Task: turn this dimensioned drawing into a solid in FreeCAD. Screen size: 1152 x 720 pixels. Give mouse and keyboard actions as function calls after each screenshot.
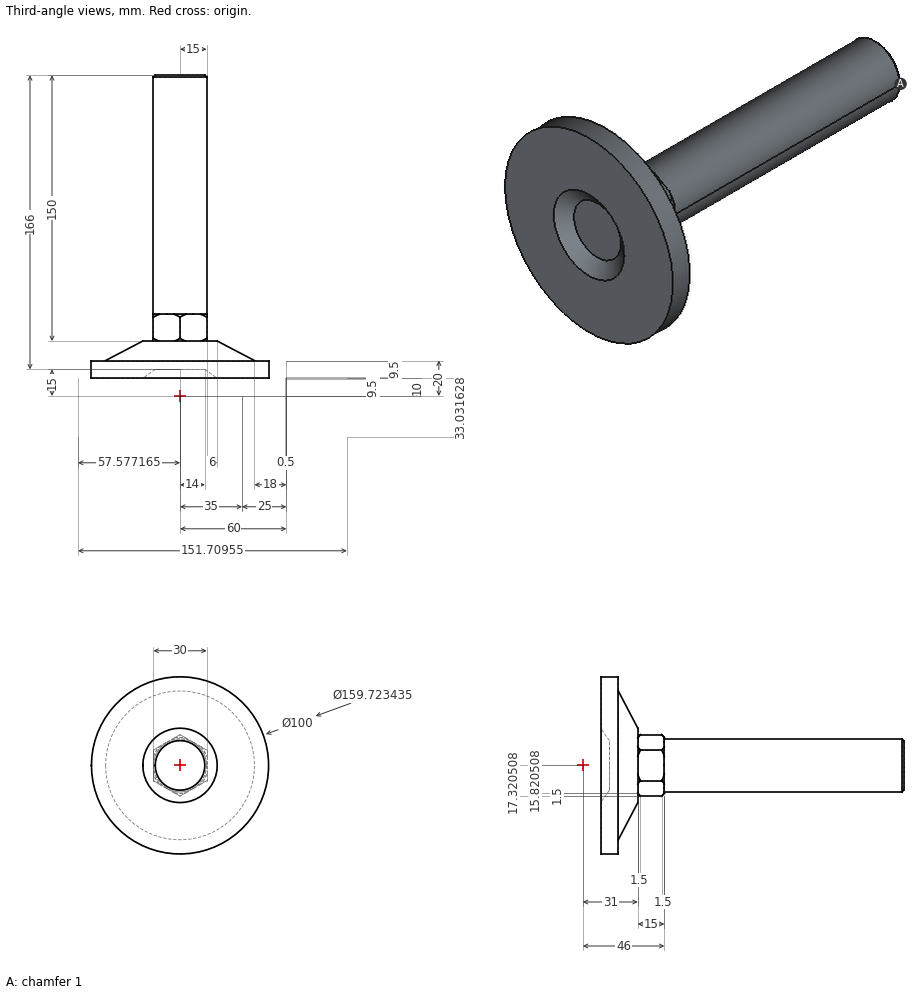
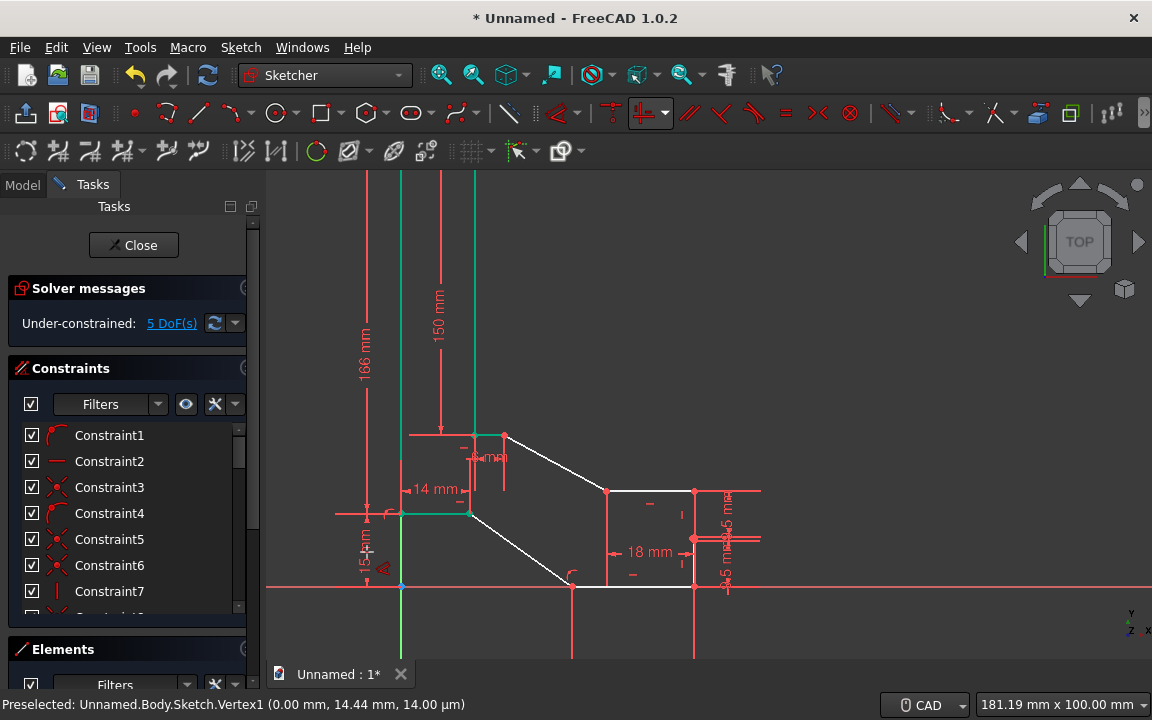
click(572, 587)
click(487, 621)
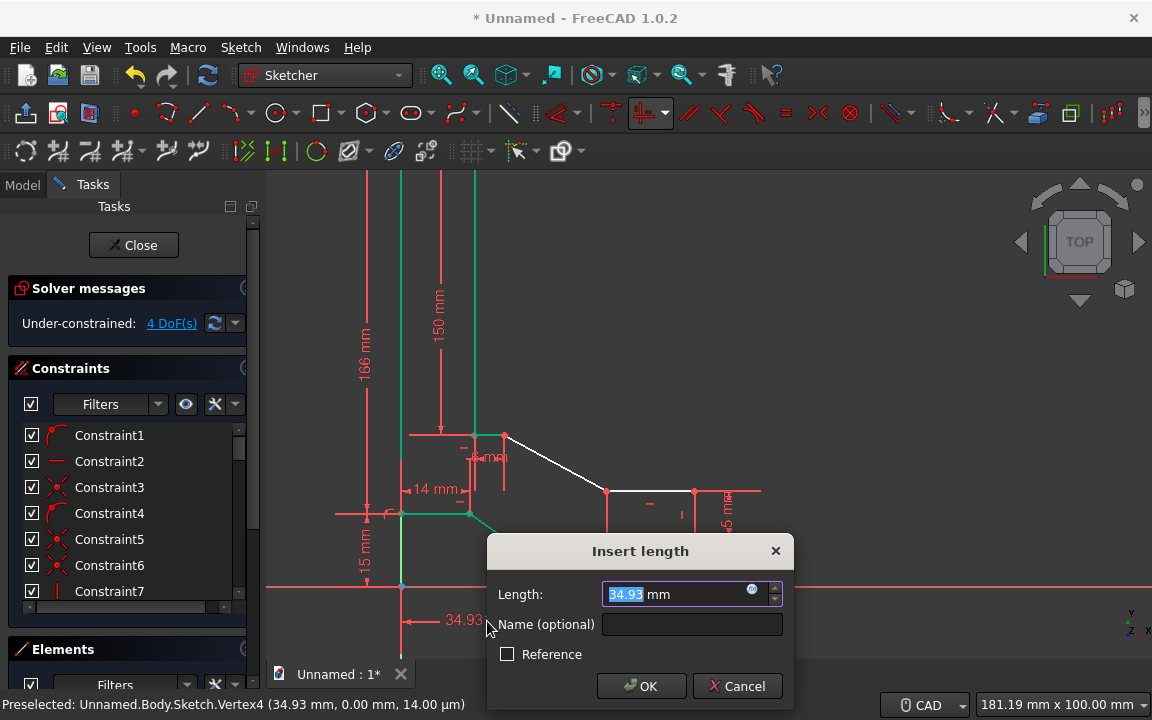
text(35)
key(Return)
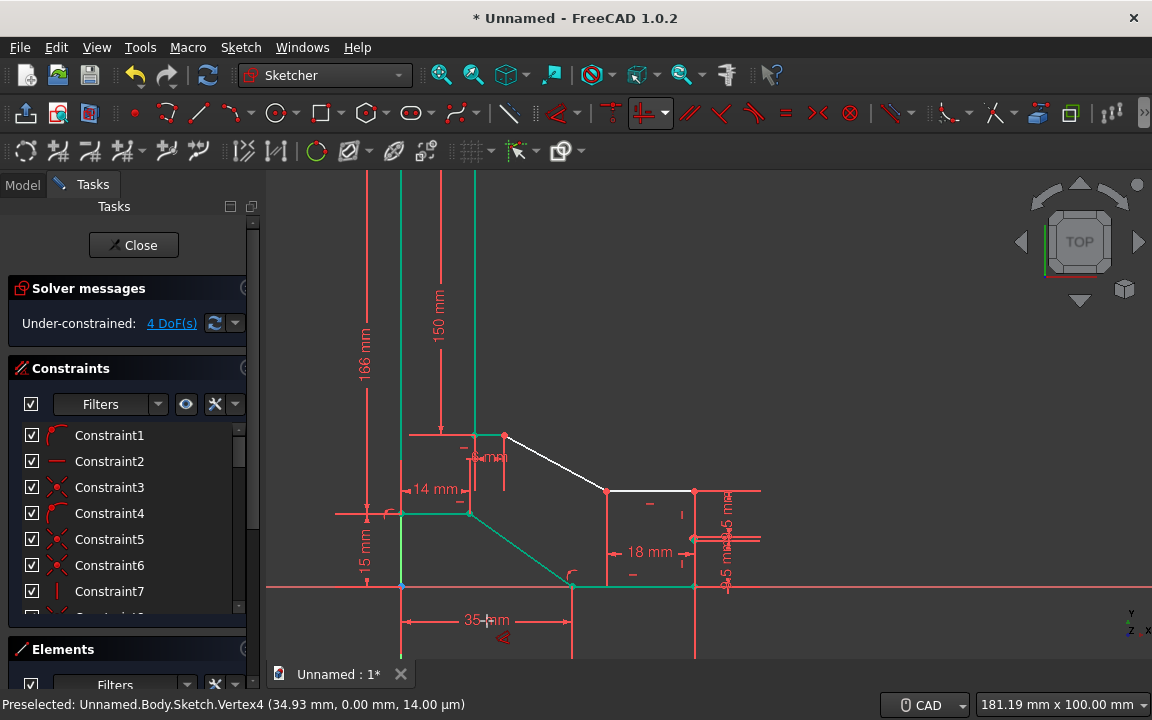
scroll(692, 538, up, 8)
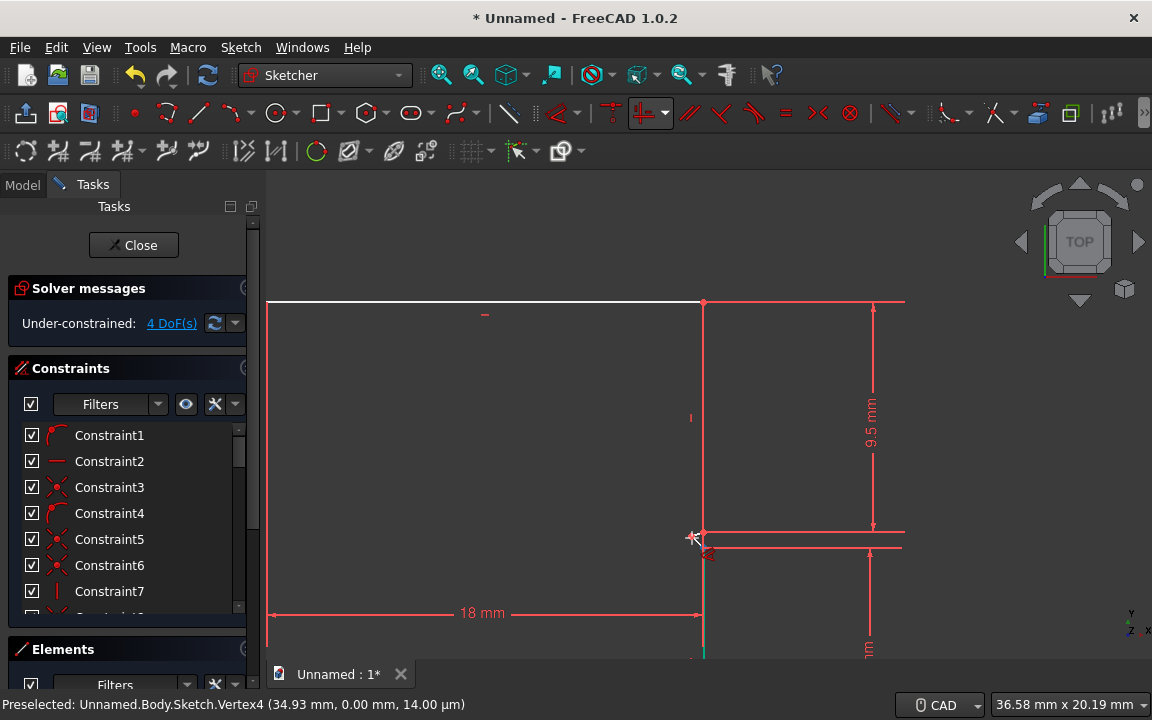
click(691, 536)
click(725, 584)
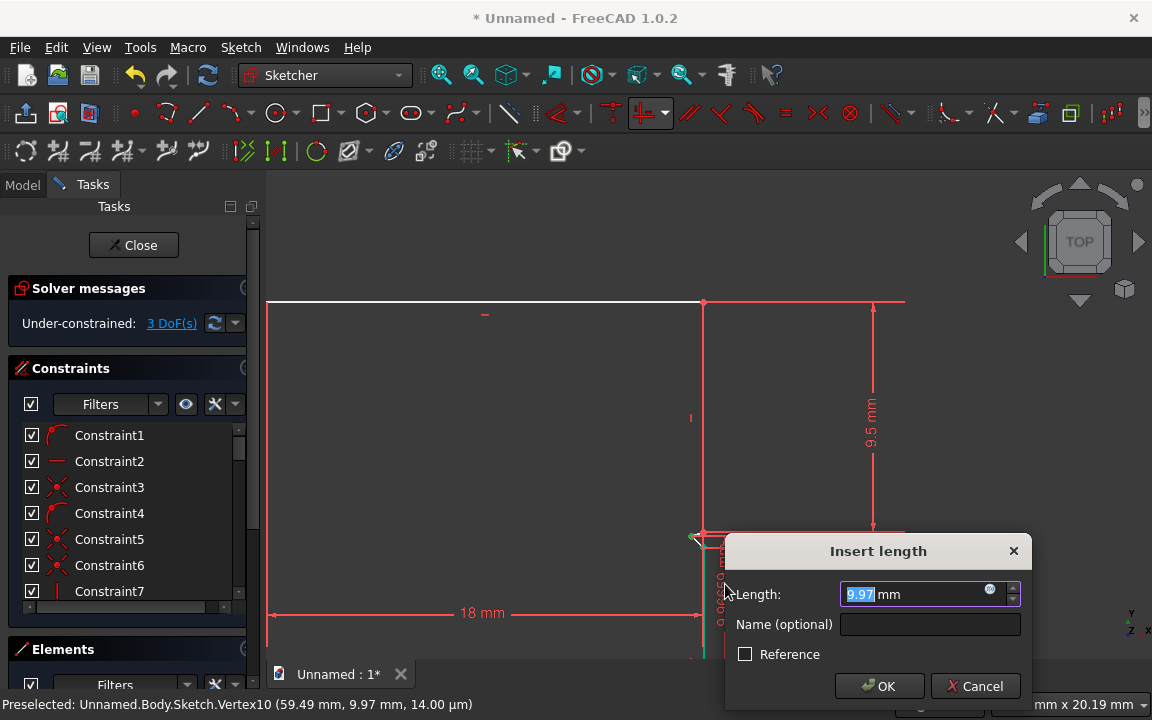
text(10)
key(Return)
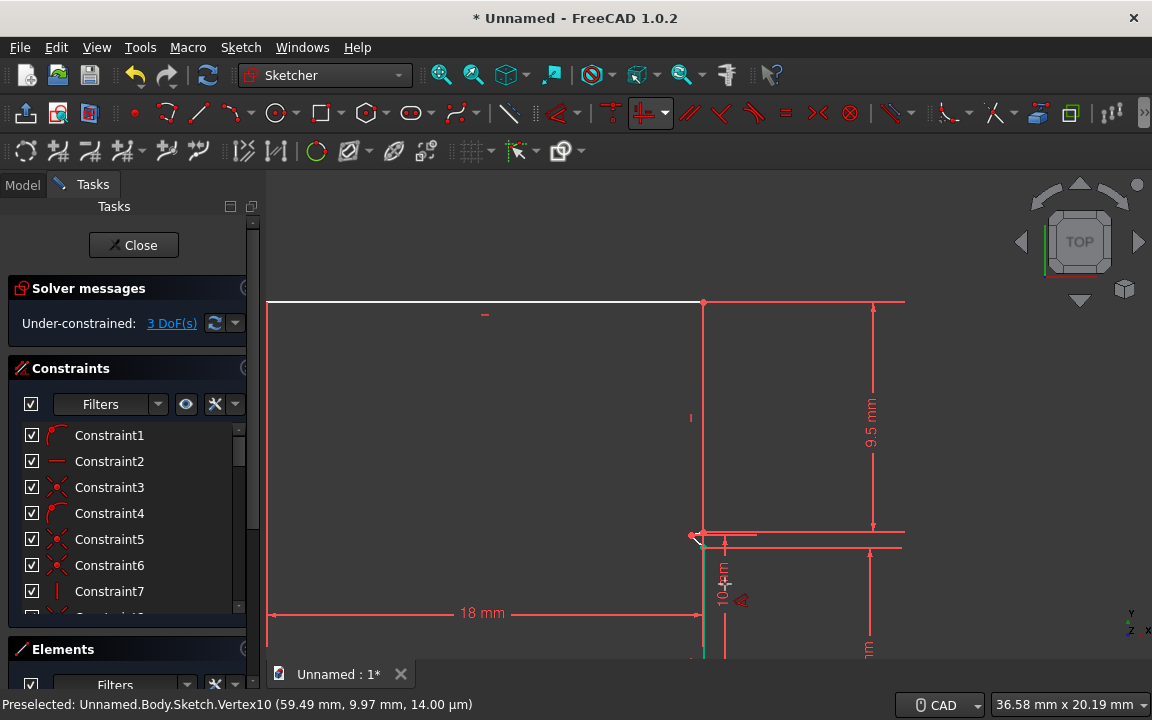
click(703, 532)
click(499, 498)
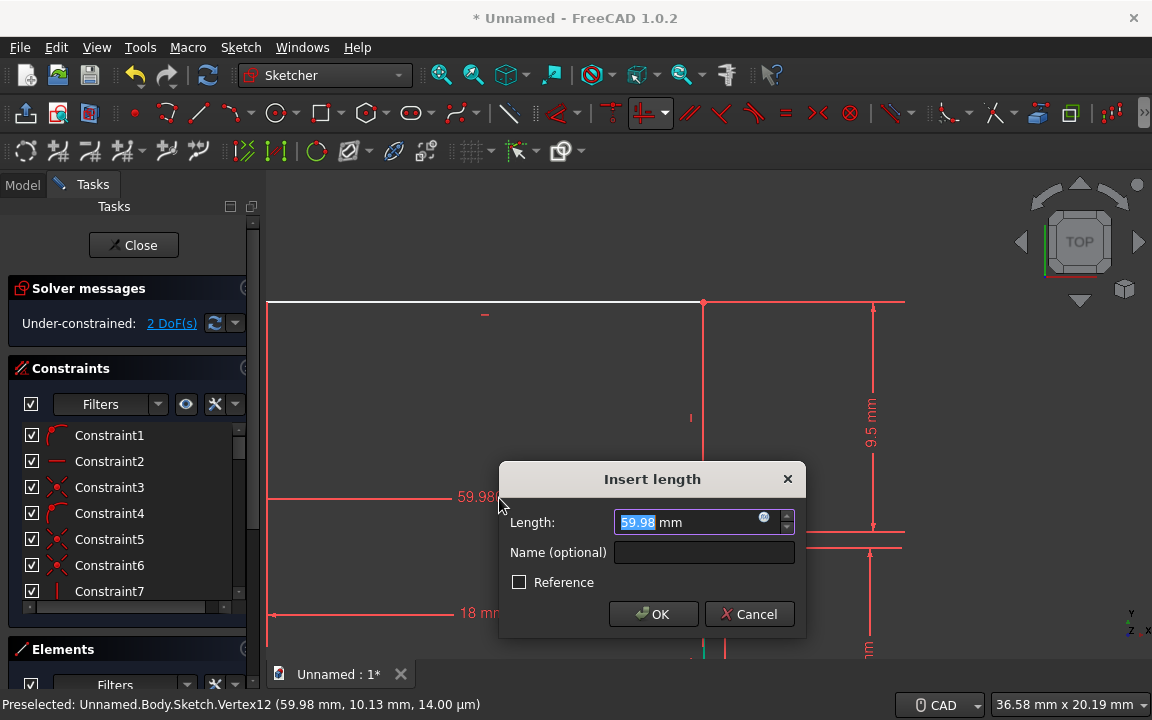
text(60)
key(Return)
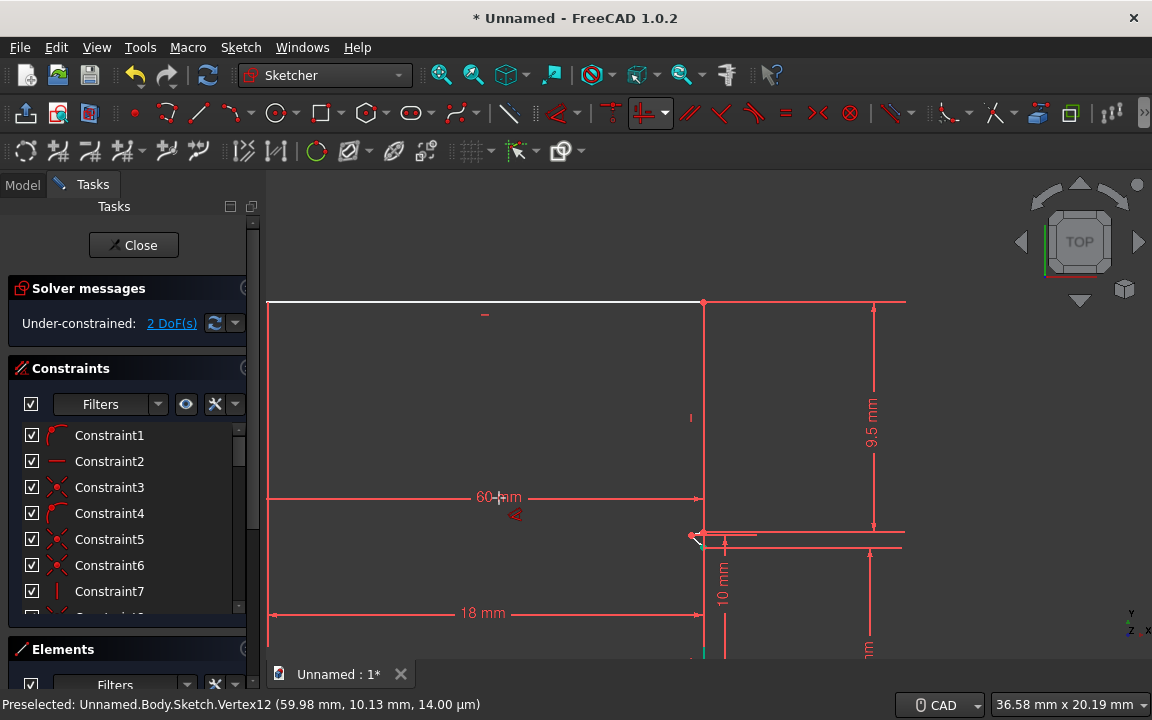
scroll(694, 561, down, 13)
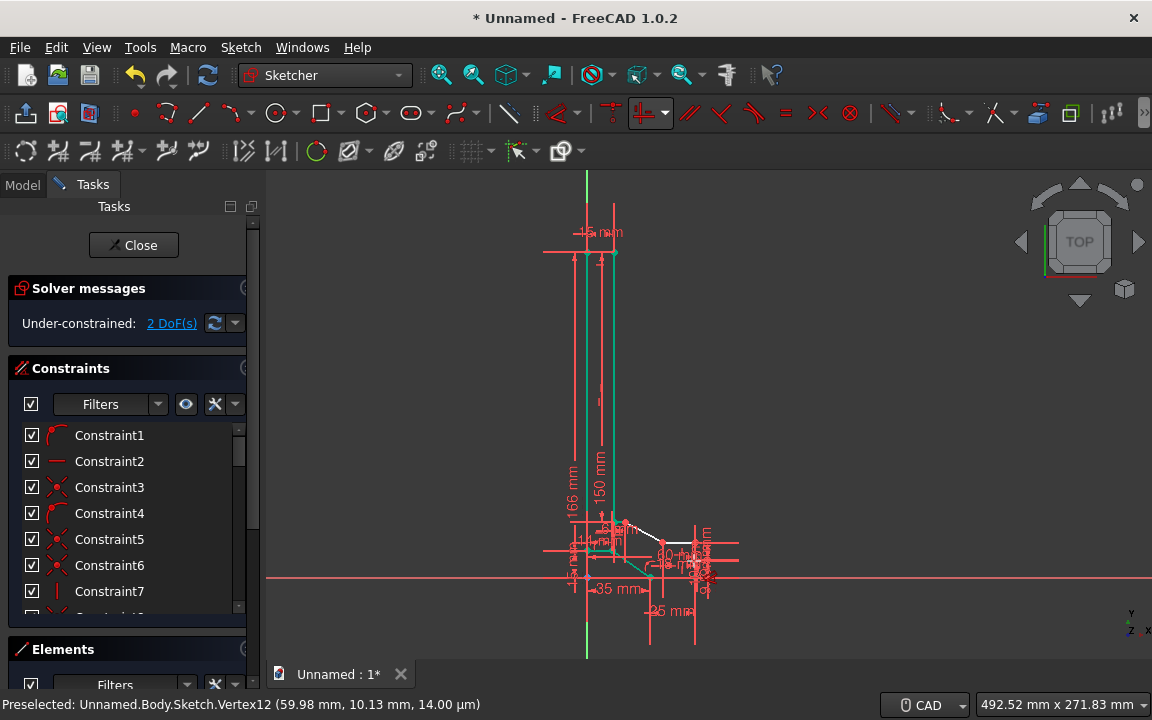
click(695, 543)
click(801, 560)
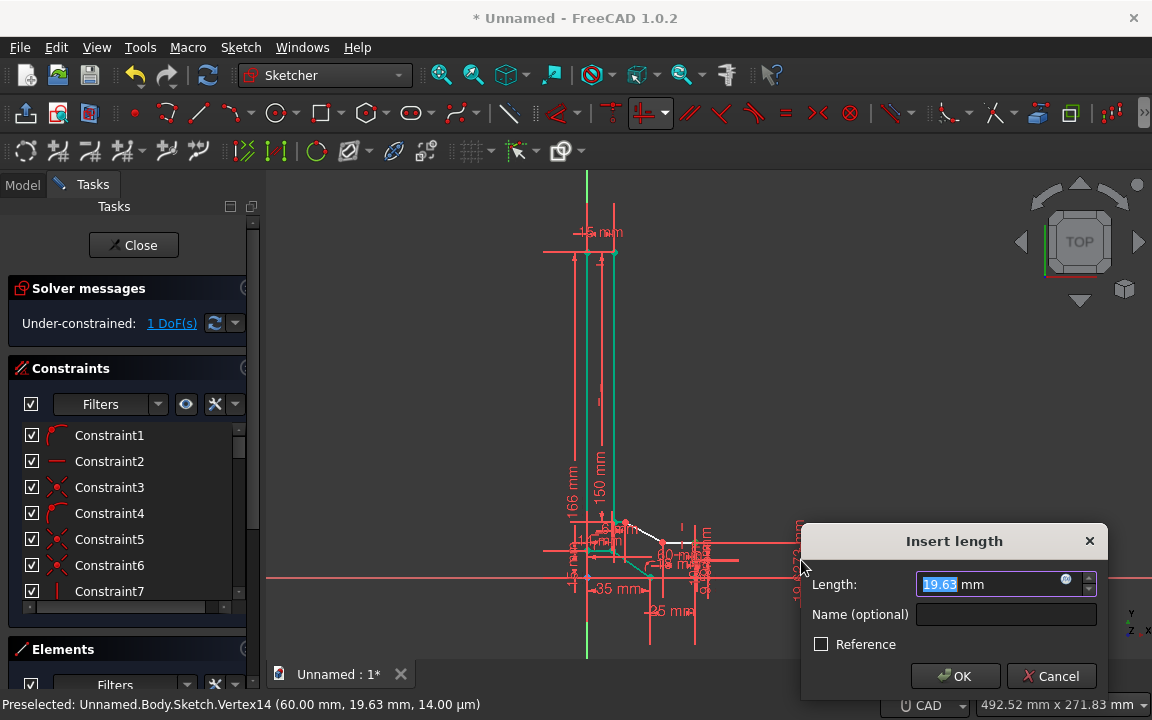
text(20)
key(Return)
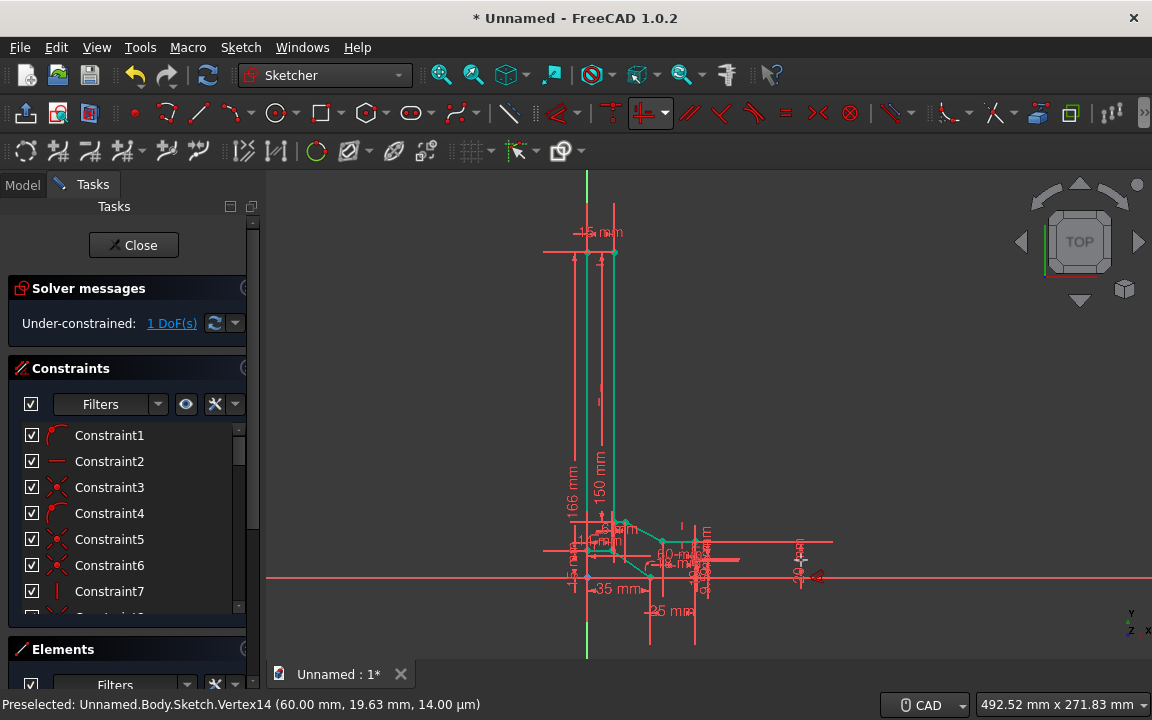
scroll(695, 560, up, 19)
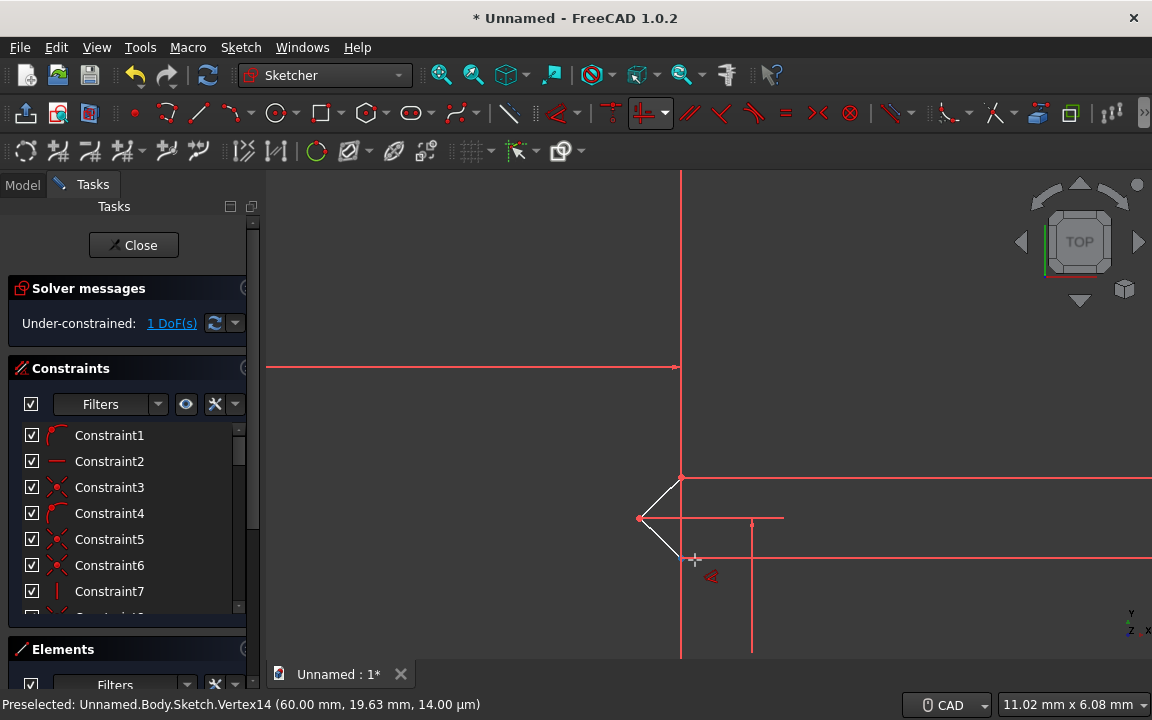
click(661, 538)
click(661, 592)